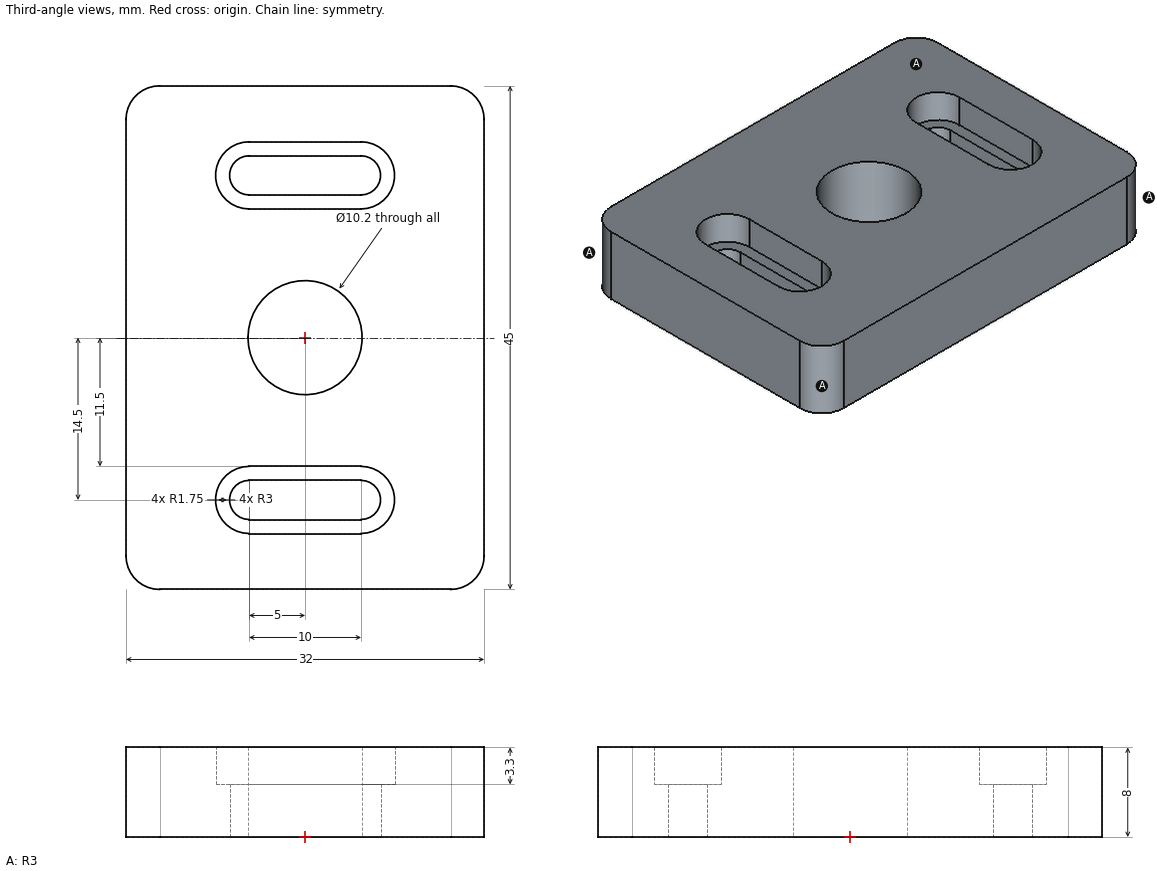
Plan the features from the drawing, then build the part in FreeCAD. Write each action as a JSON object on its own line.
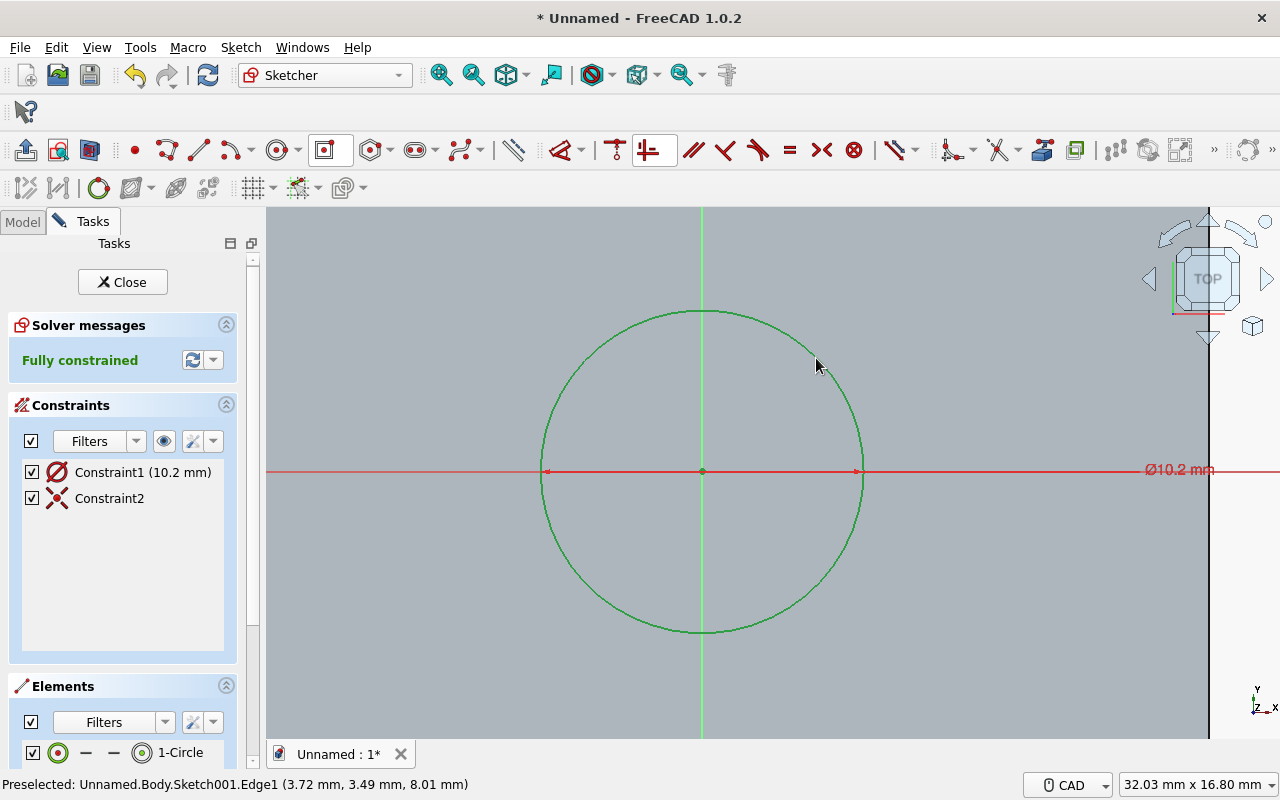
{"action": "left_click", "coordinate": [123, 282]}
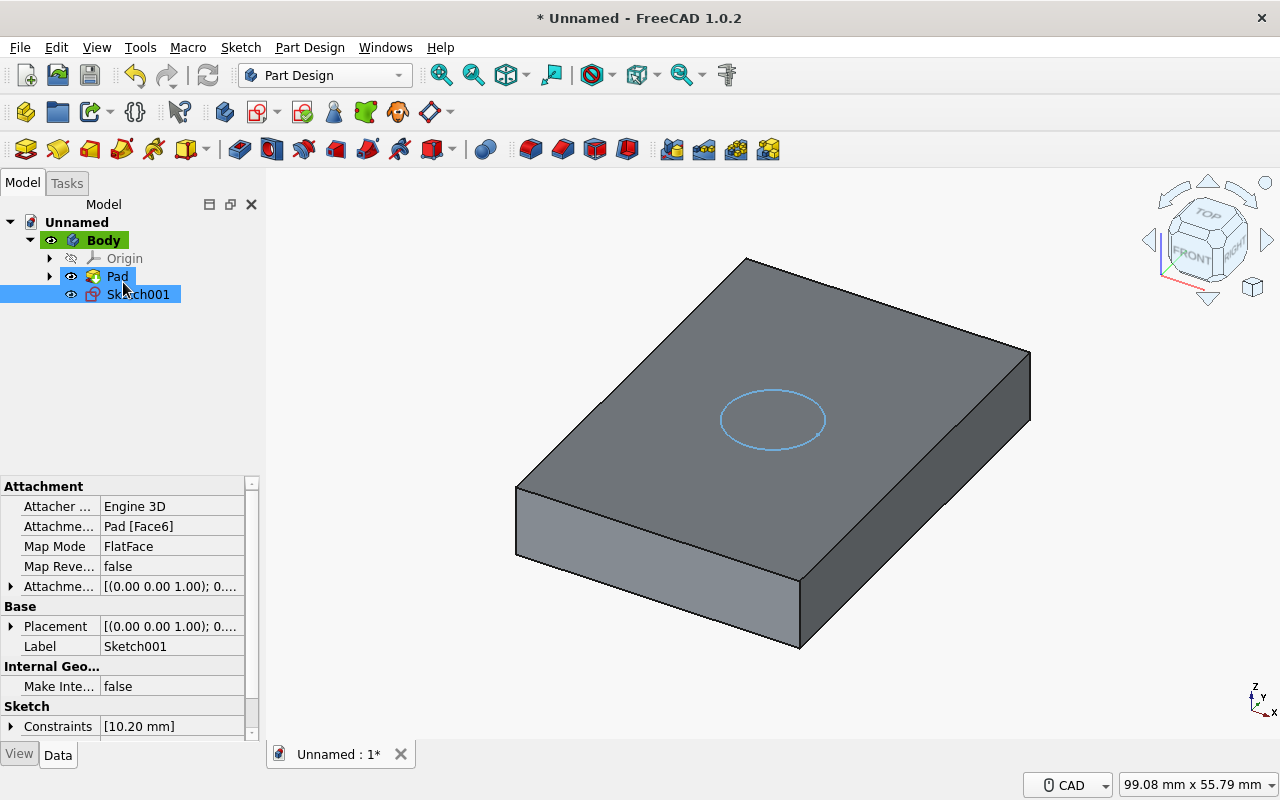
{"action": "left_click", "coordinate": [272, 150]}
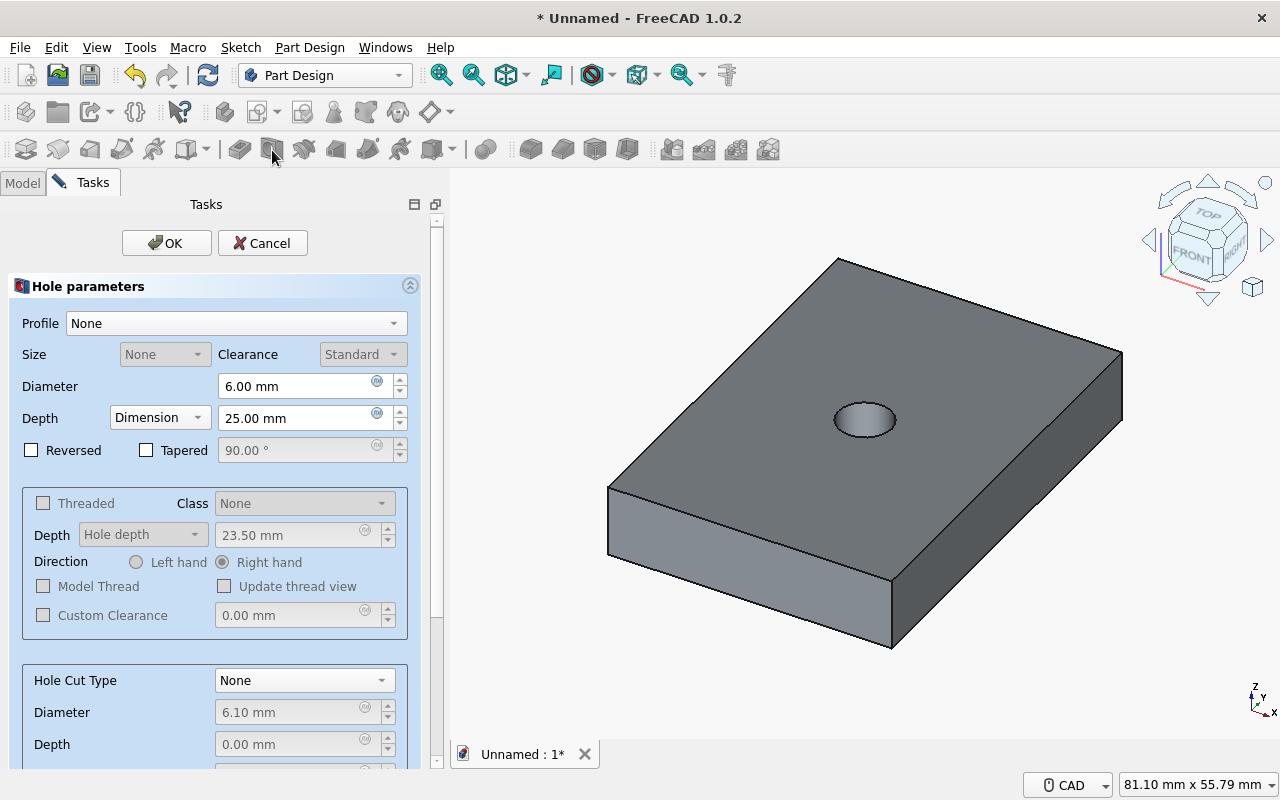
{"action": "triple_click", "coordinate": [305, 386]}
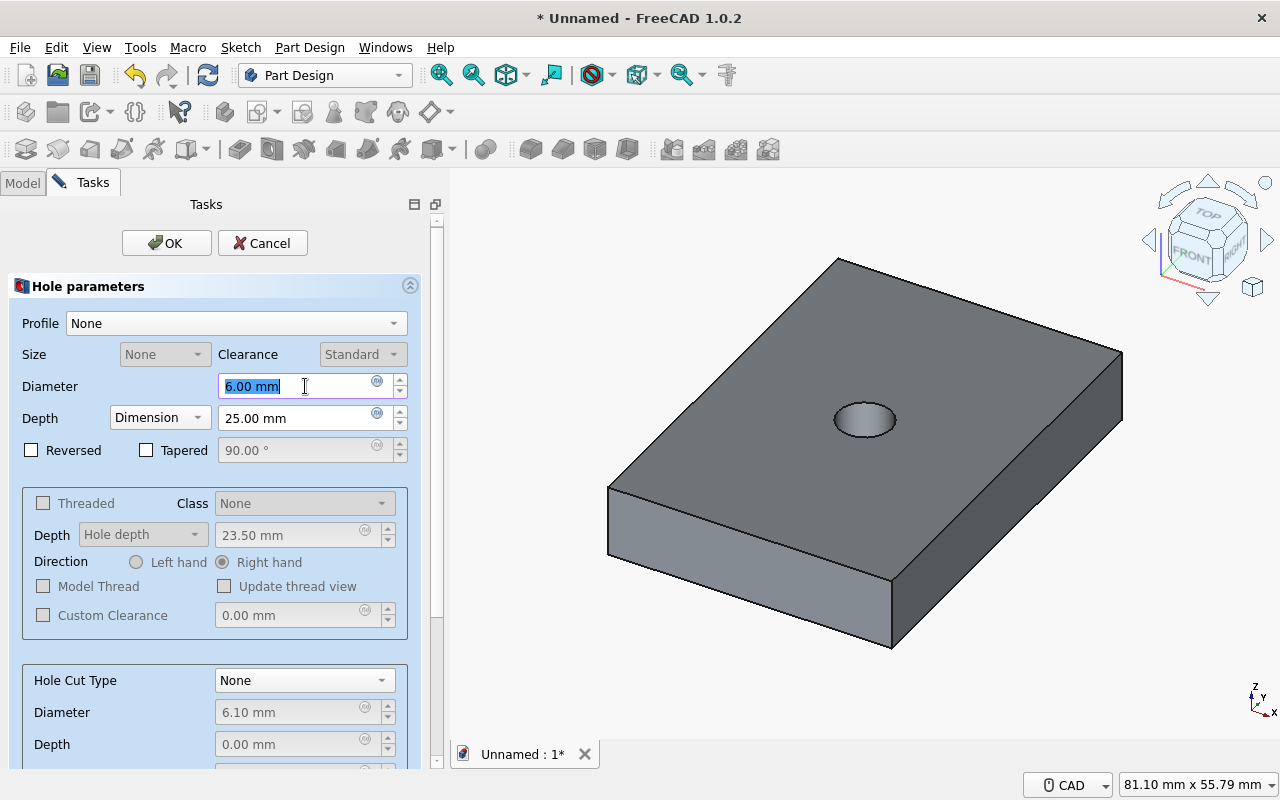
{"action": "type", "text": "10.2"}
{"action": "key", "text": "Tab"}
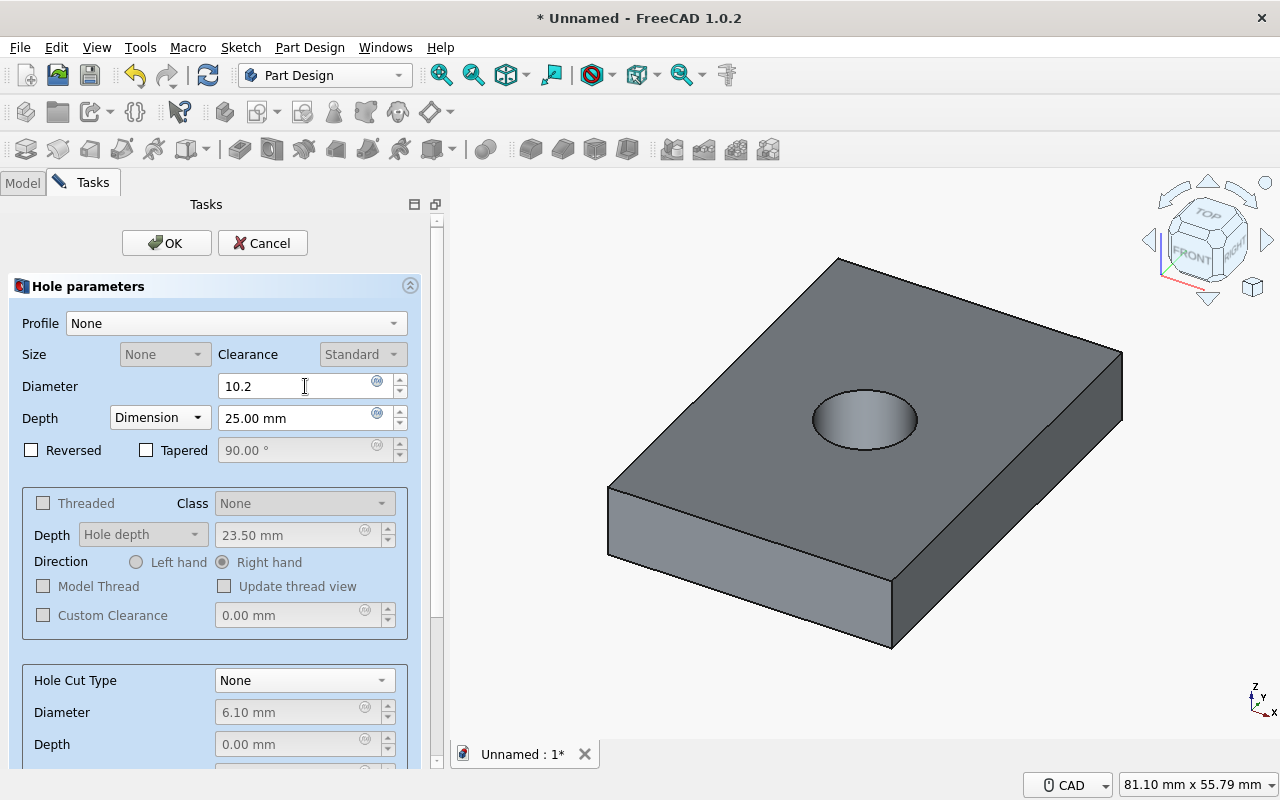
{"action": "left_click", "coordinate": [161, 418]}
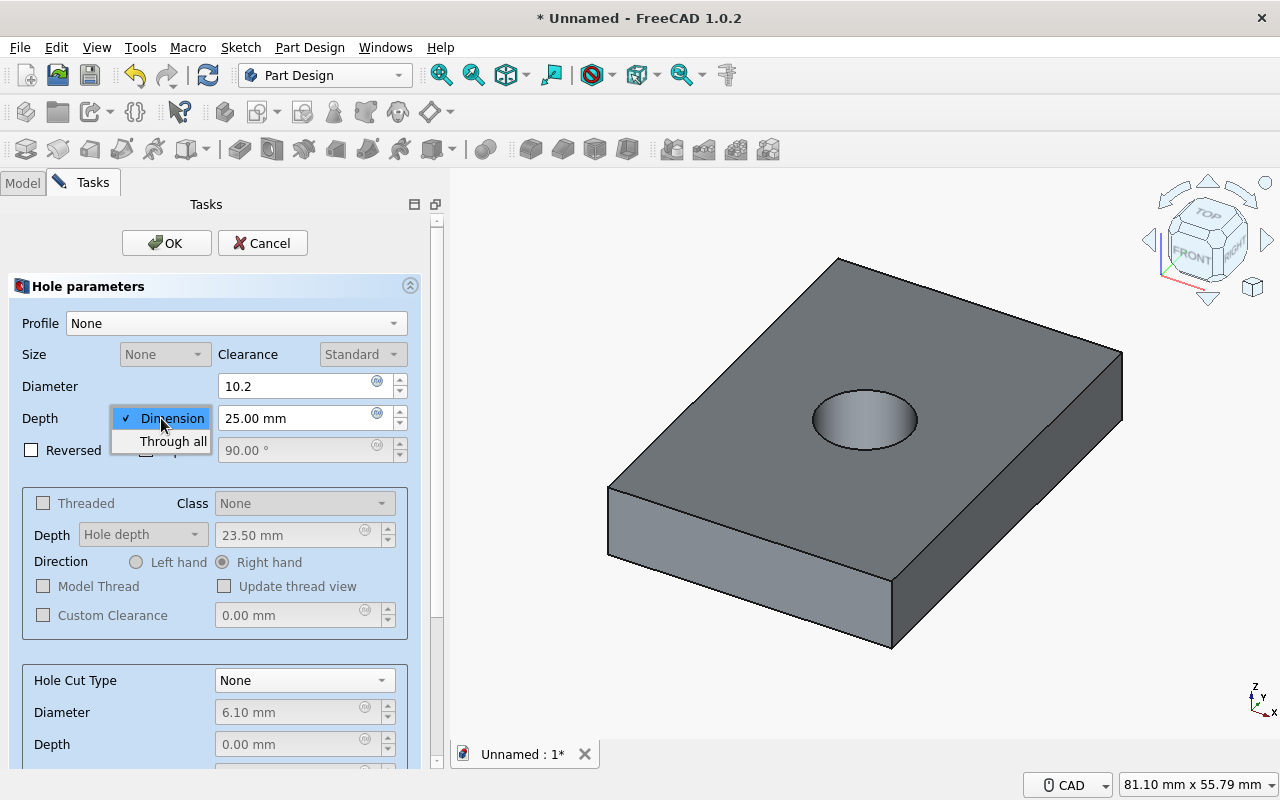
{"action": "left_click", "coordinate": [160, 442]}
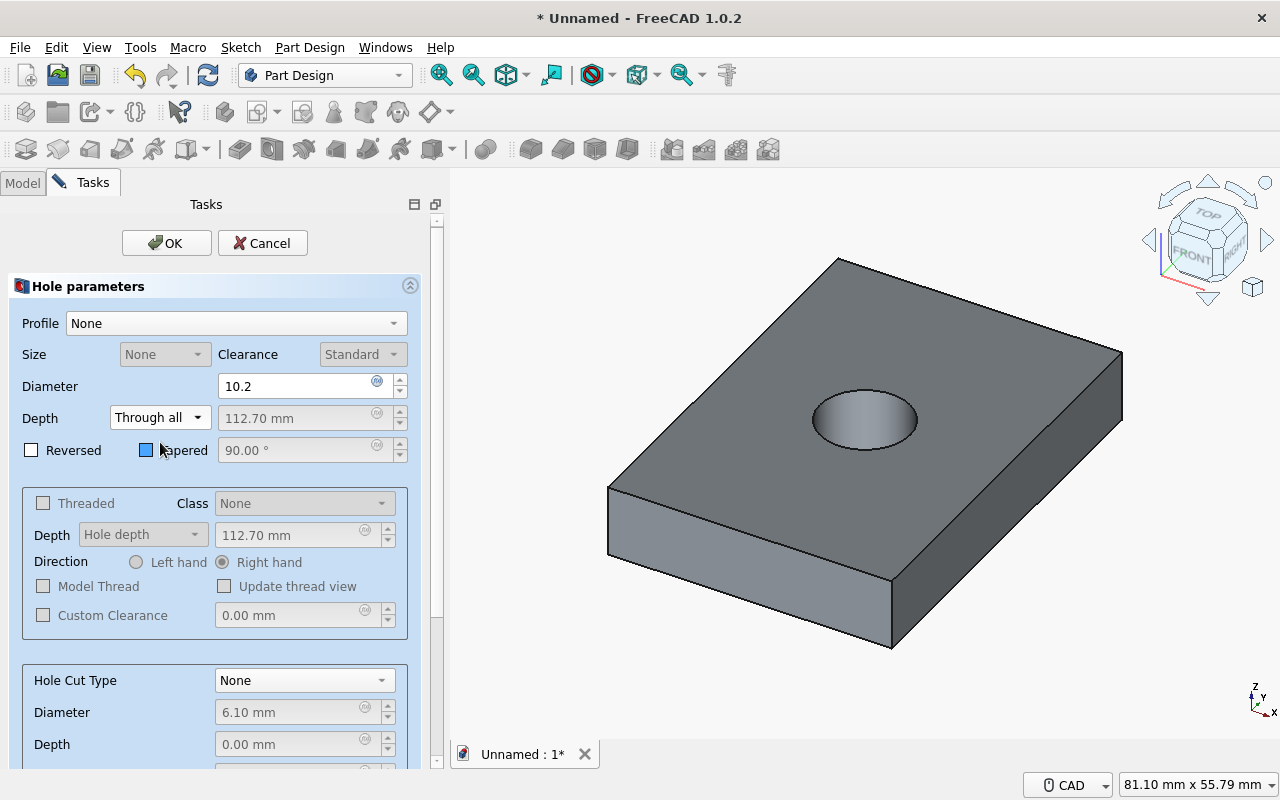
{"action": "left_click", "coordinate": [167, 243]}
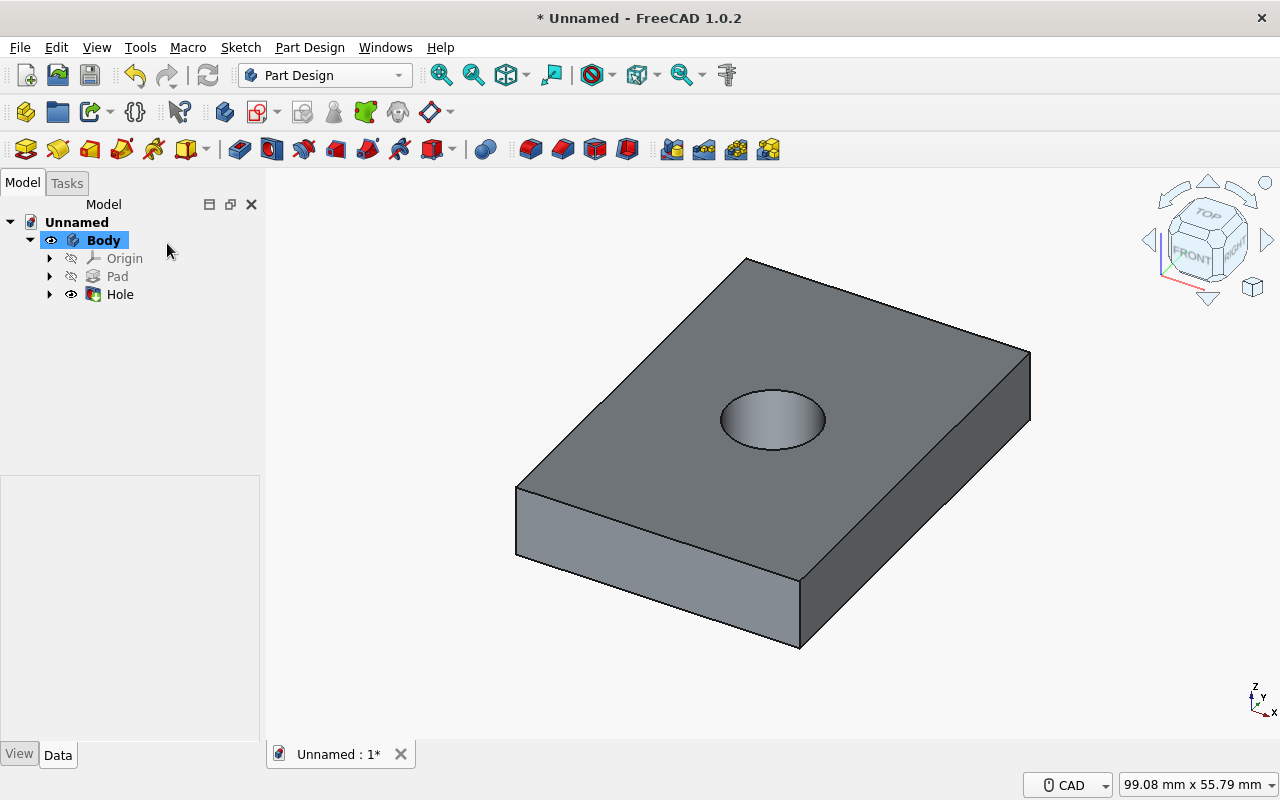
{"action": "left_click", "coordinate": [748, 498]}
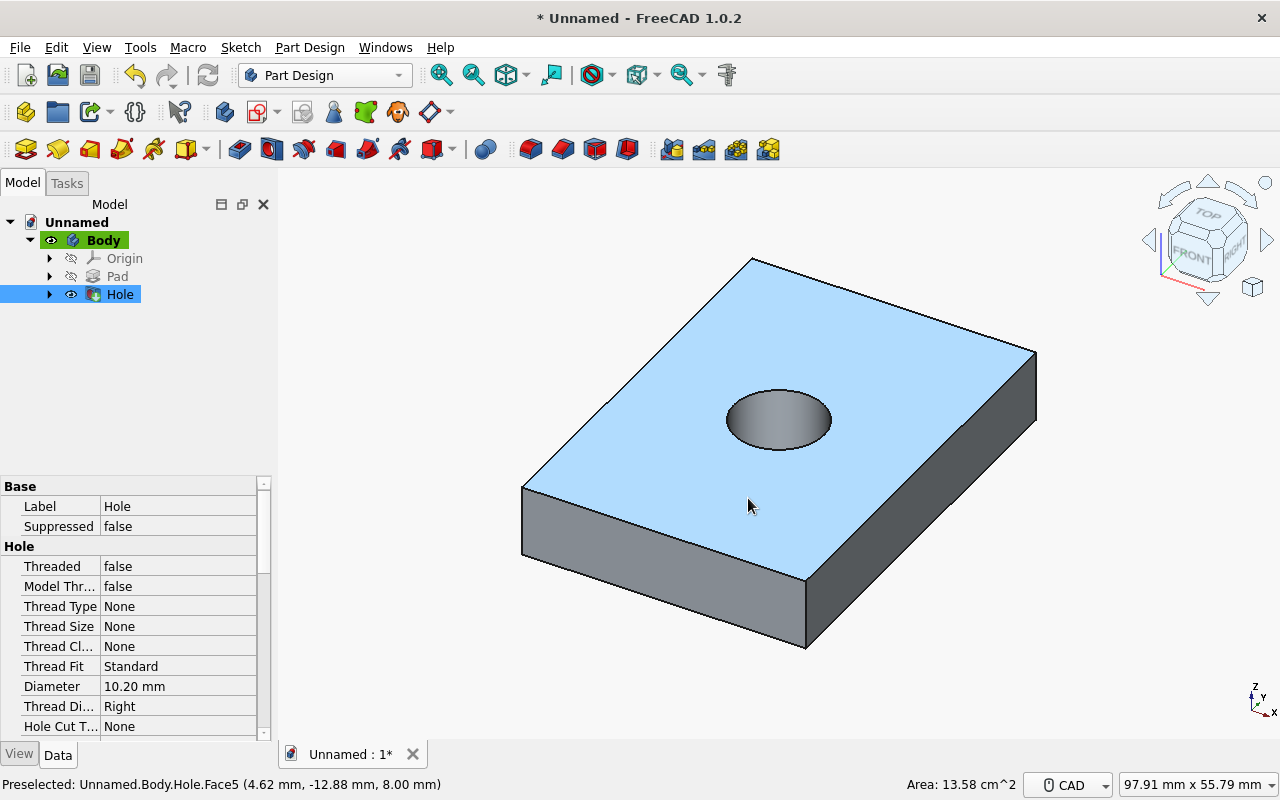
{"action": "left_click", "coordinate": [258, 112]}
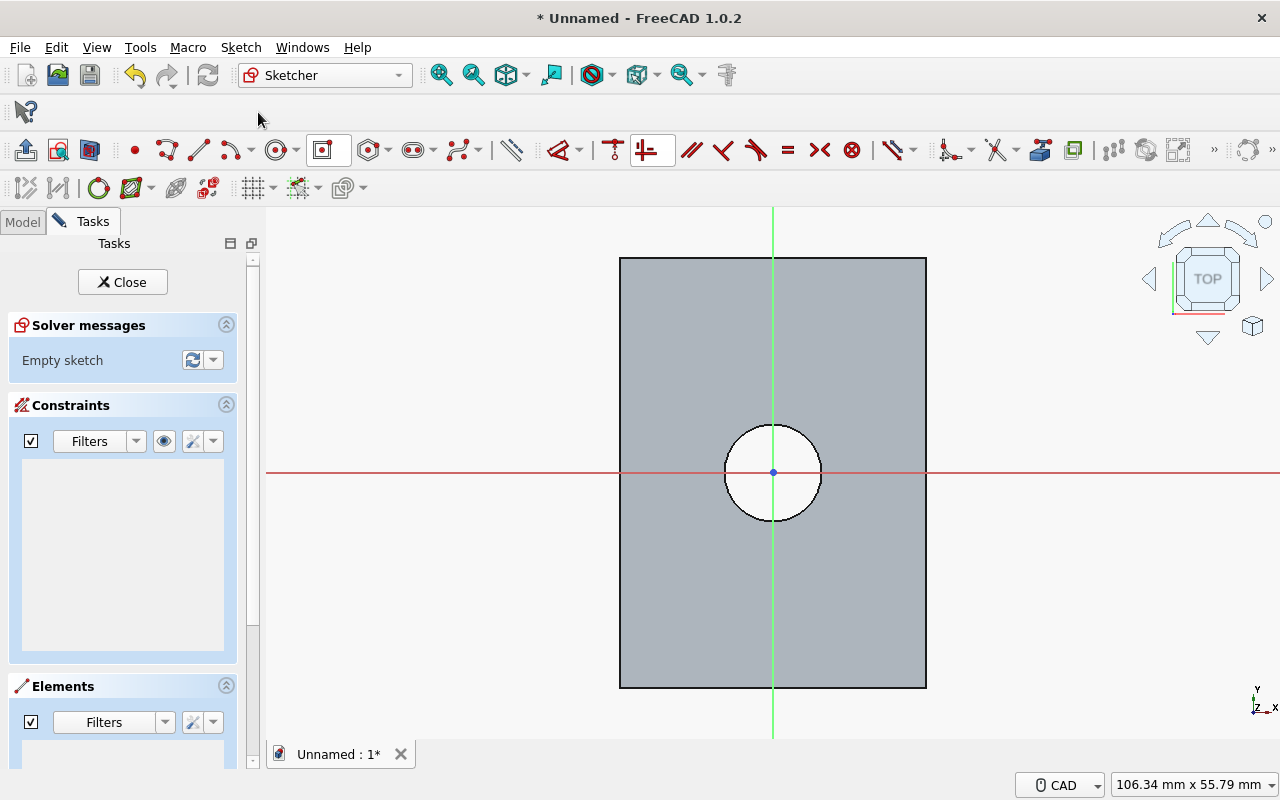
{"action": "left_click", "coordinate": [414, 150]}